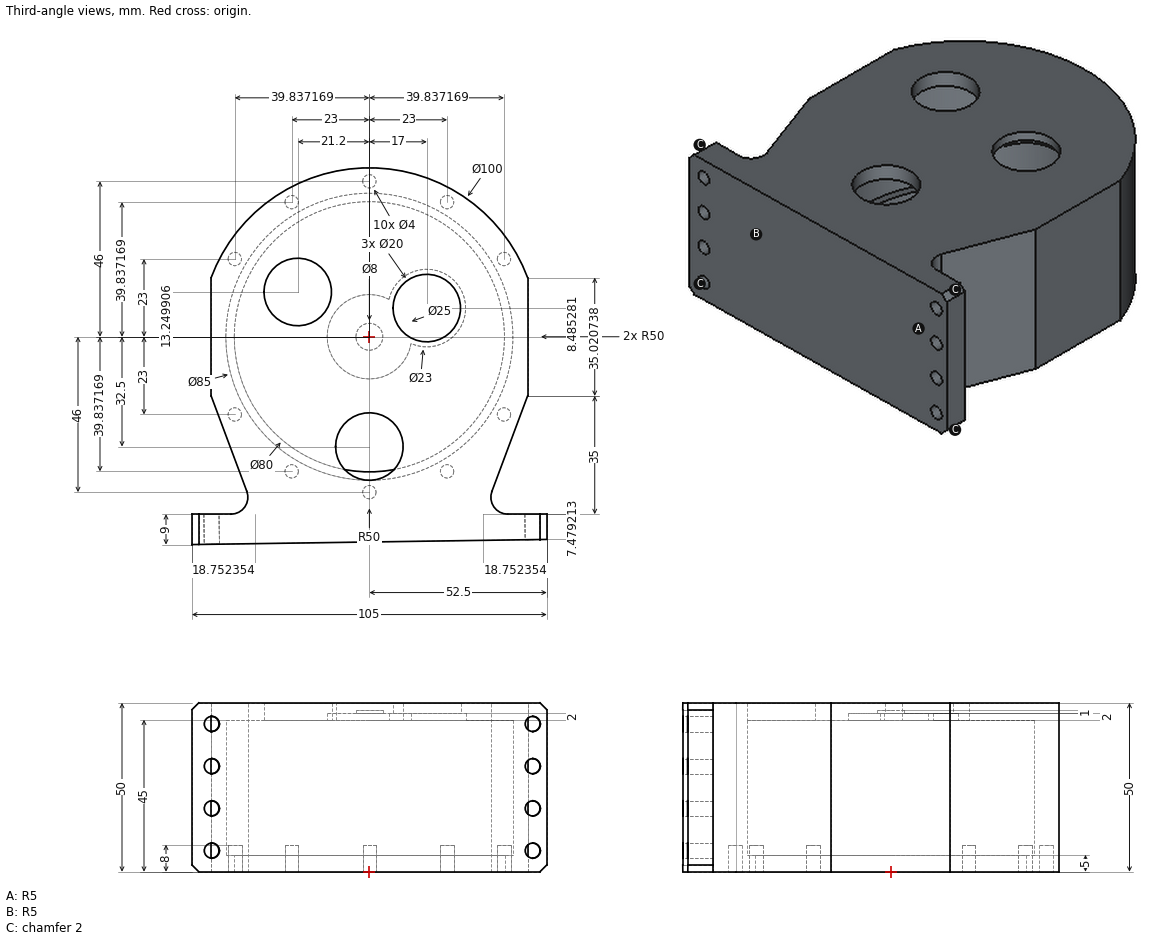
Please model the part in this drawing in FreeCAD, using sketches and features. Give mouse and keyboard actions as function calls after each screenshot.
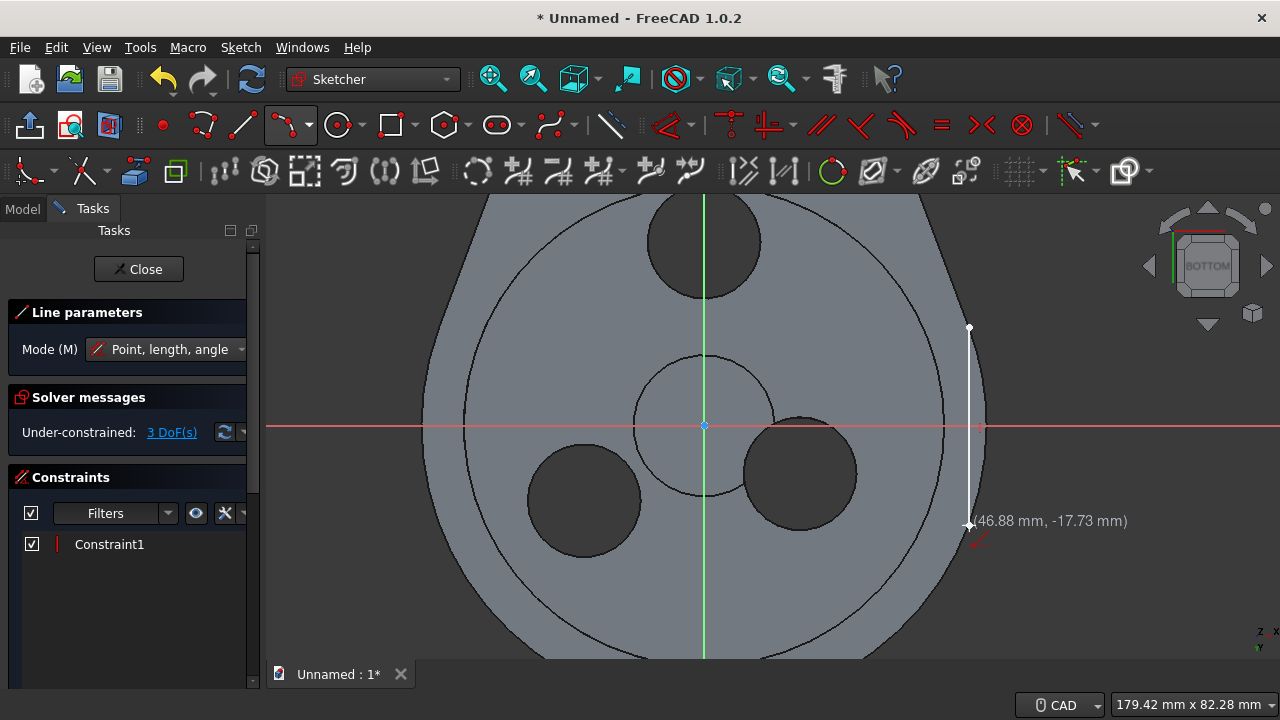
click(284, 126)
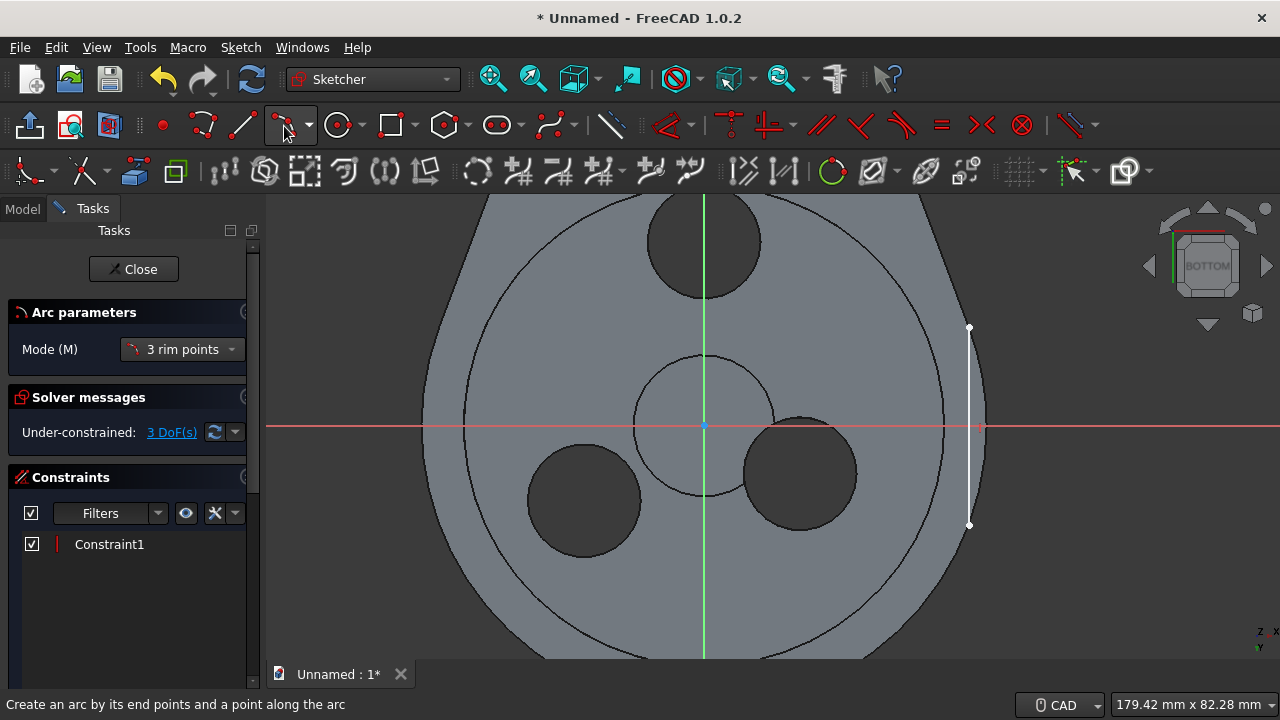
click(969, 526)
click(969, 328)
click(986, 446)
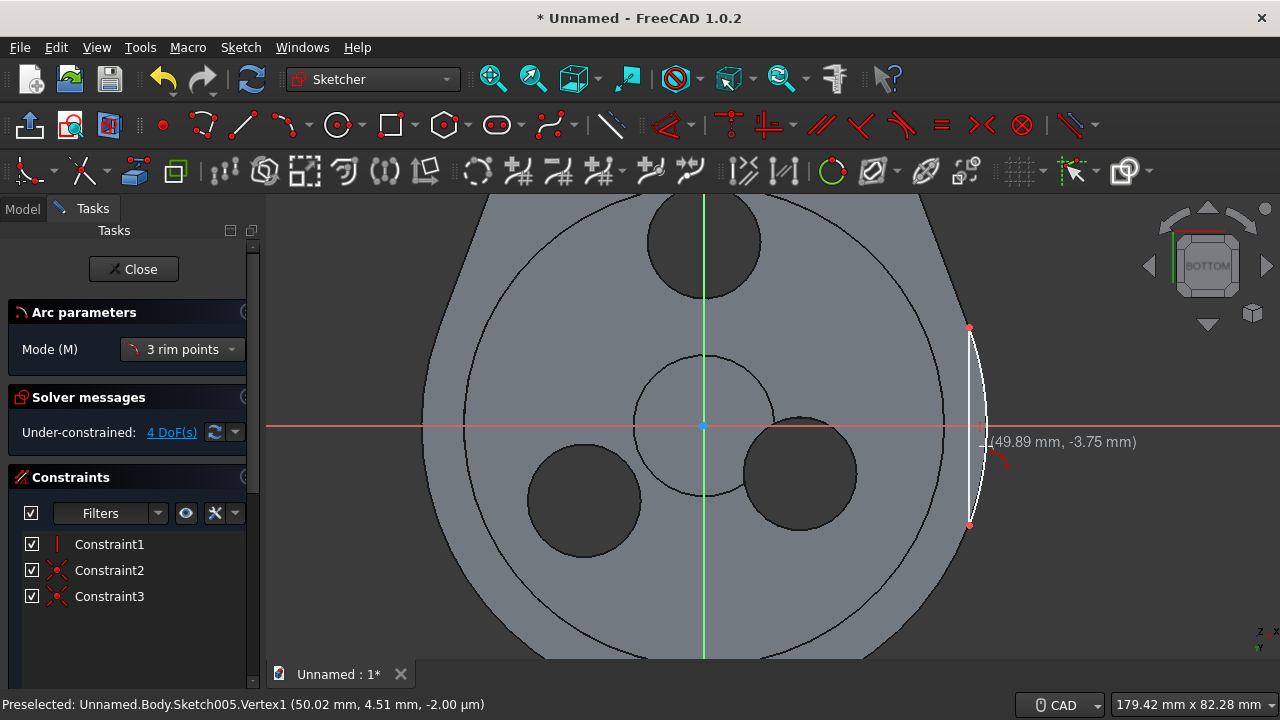
click(244, 126)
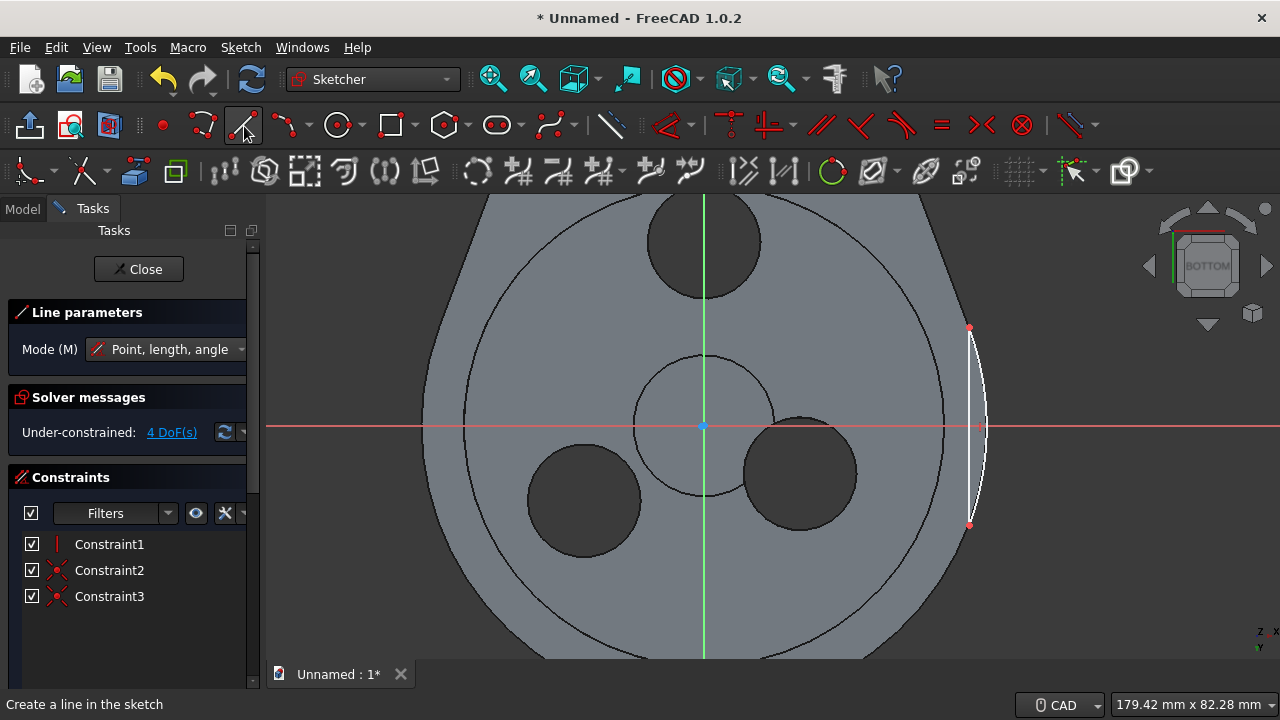
click(439, 525)
click(439, 327)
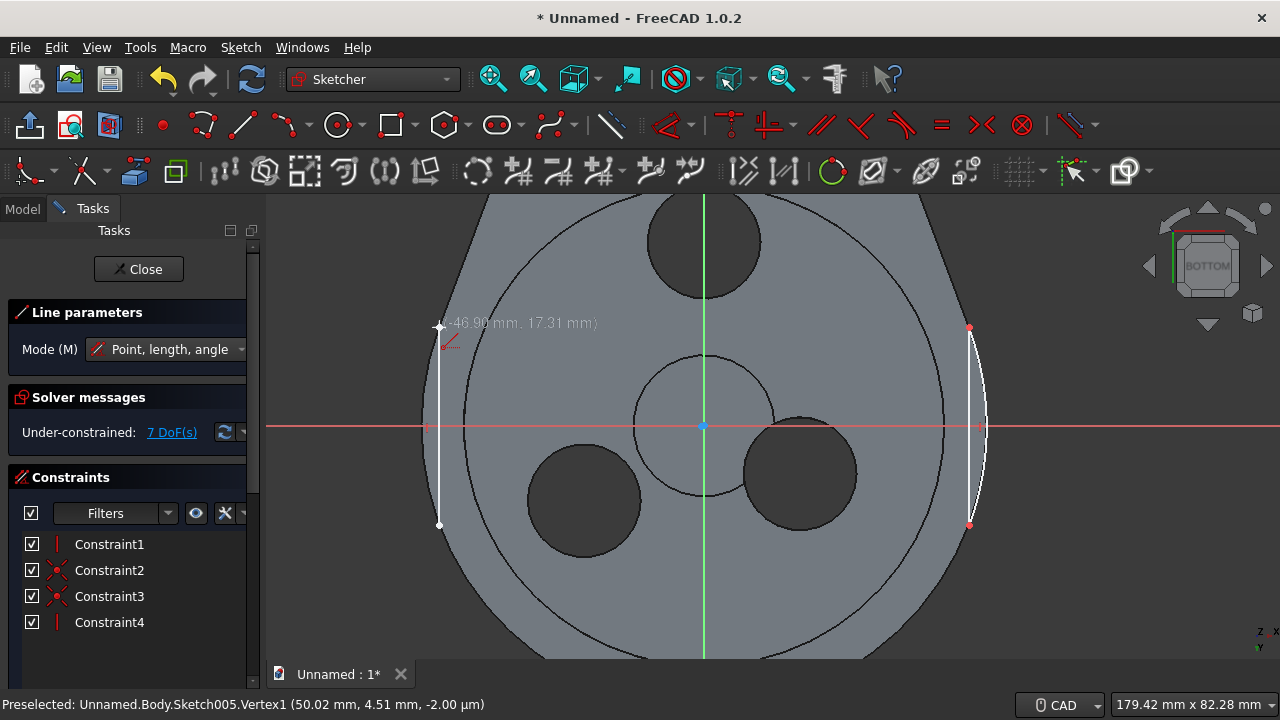
click(284, 126)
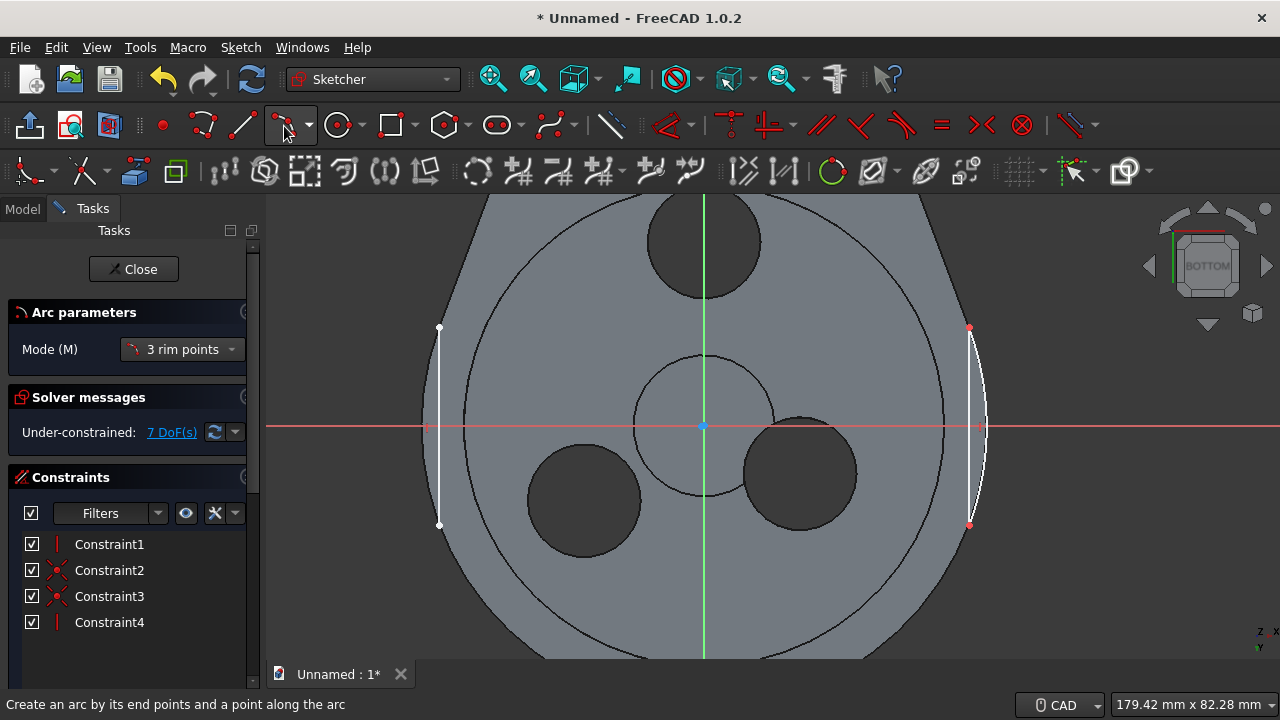
click(439, 328)
click(439, 526)
click(422, 406)
key(Escape)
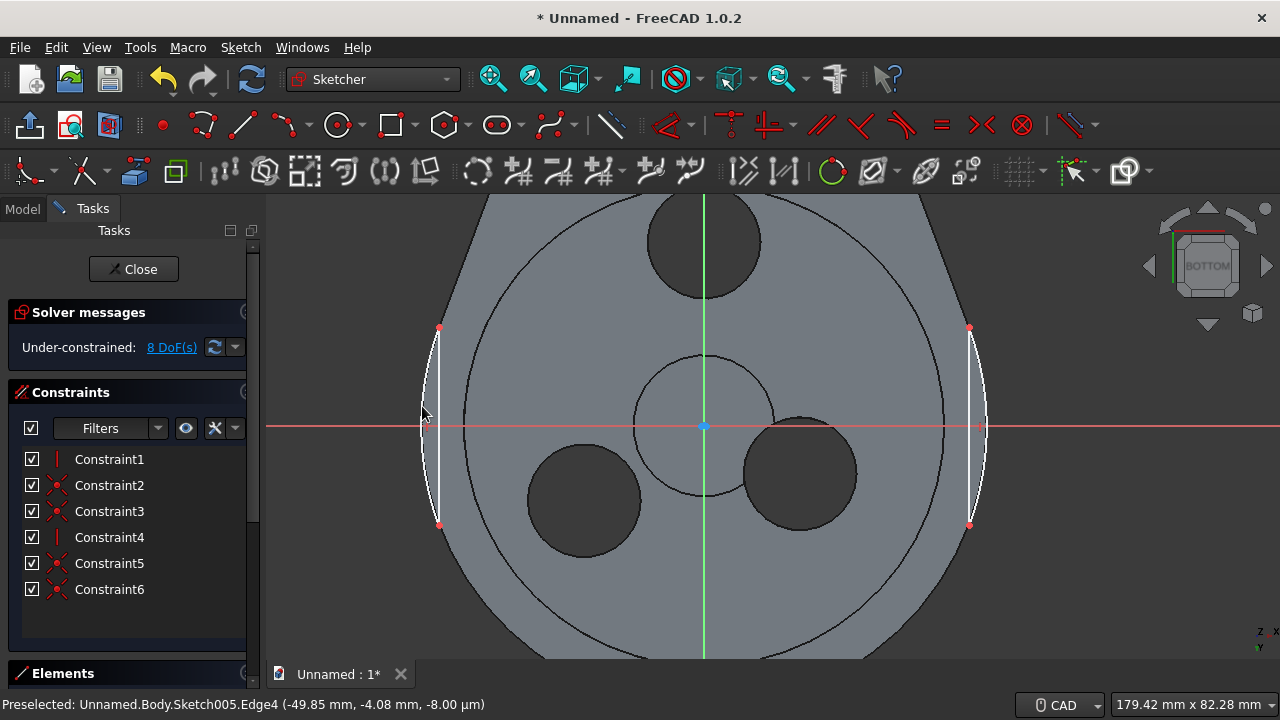
click(984, 467)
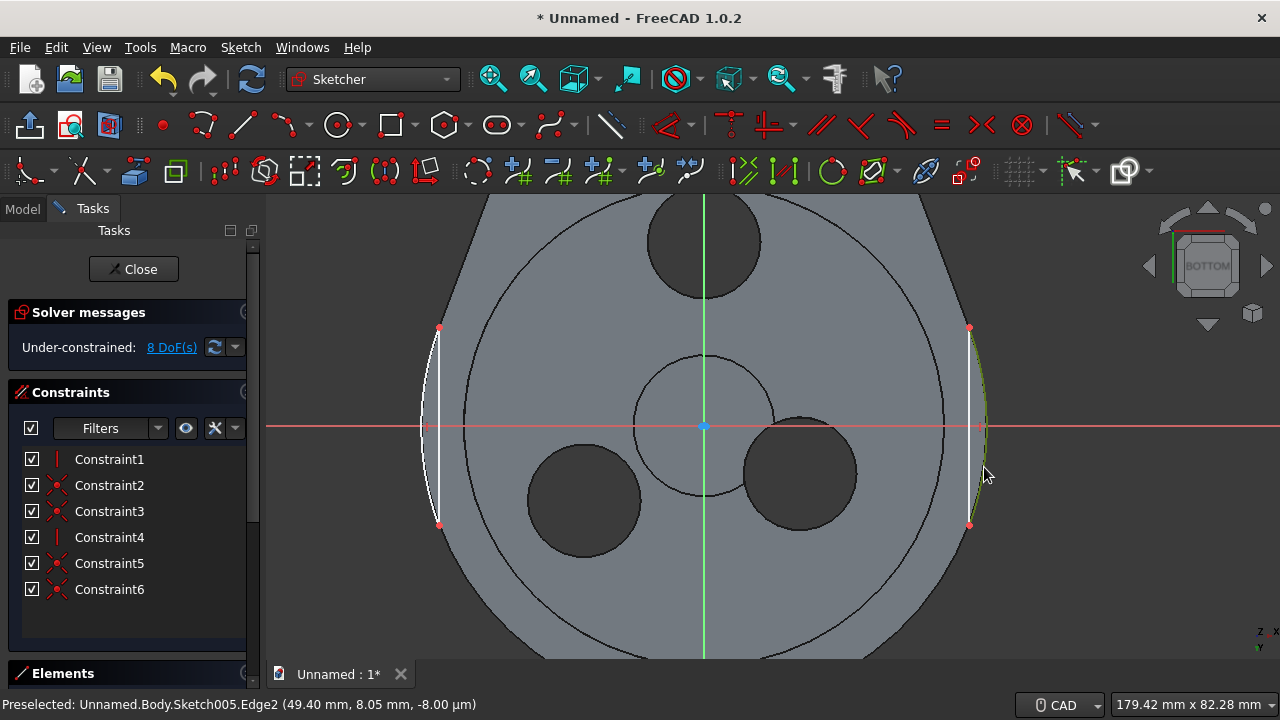
click(424, 387)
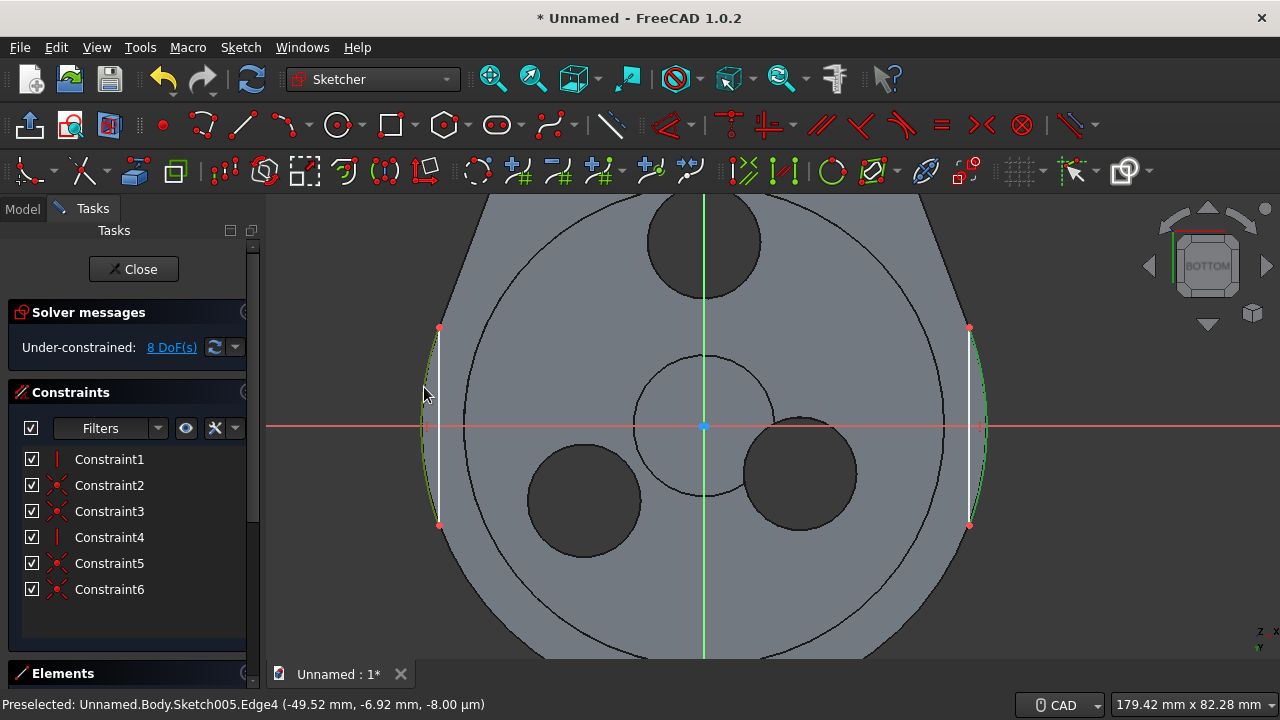
click(730, 126)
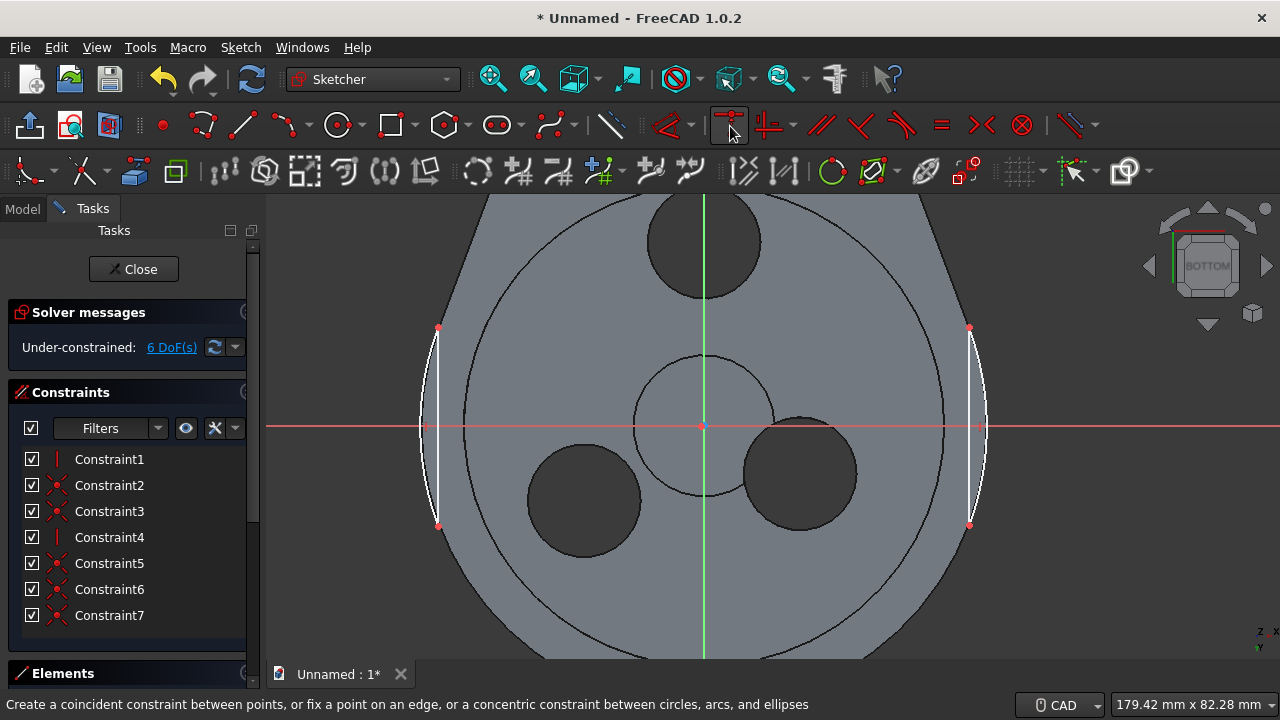
drag(692, 416, 714, 437)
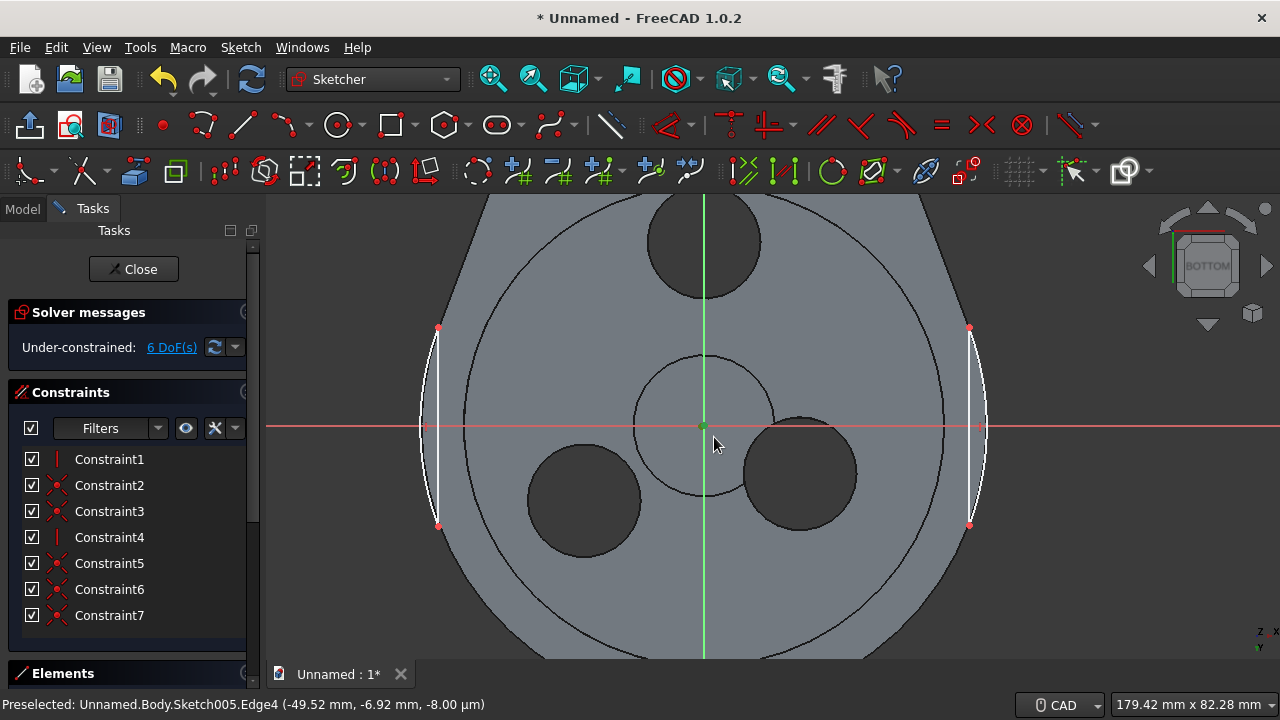
click(730, 126)